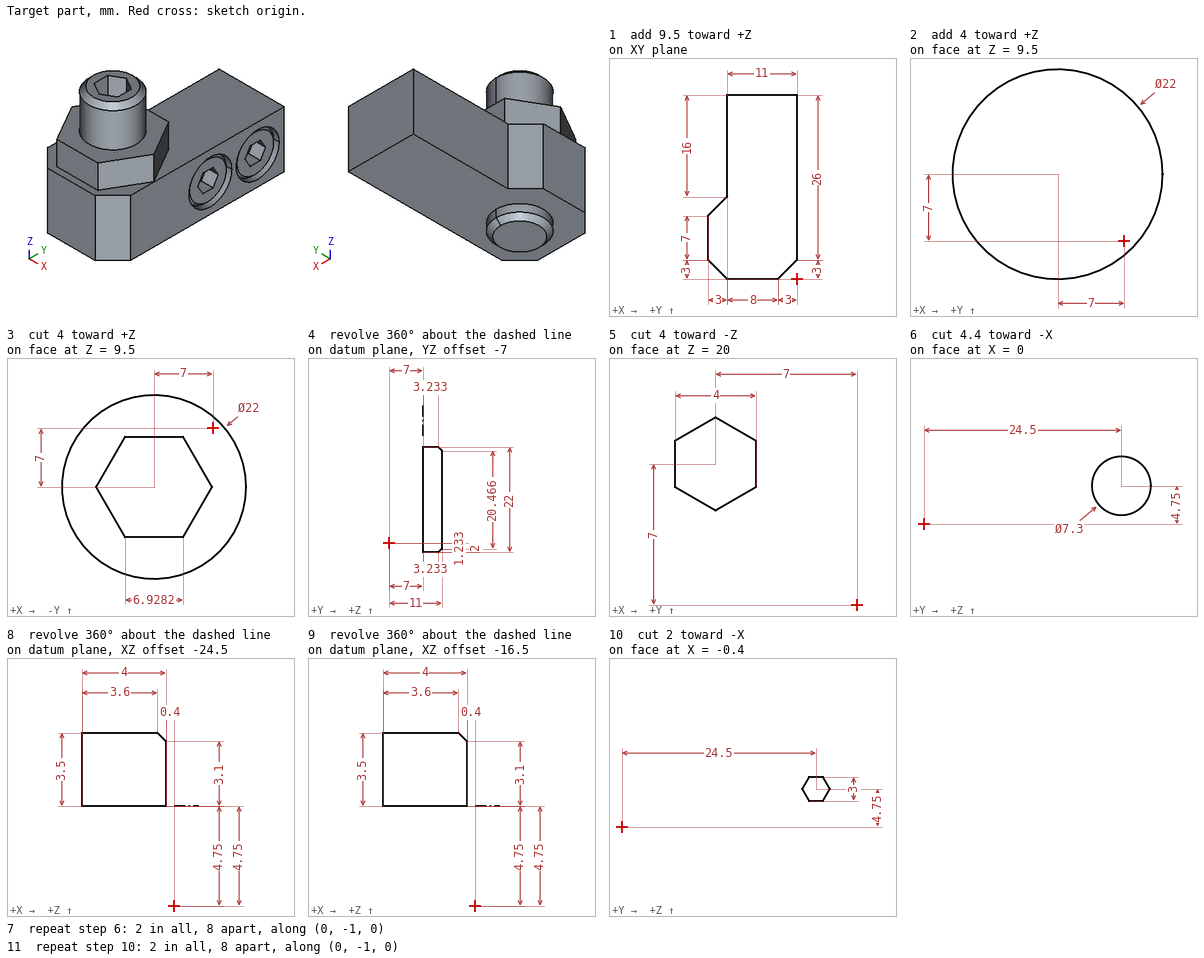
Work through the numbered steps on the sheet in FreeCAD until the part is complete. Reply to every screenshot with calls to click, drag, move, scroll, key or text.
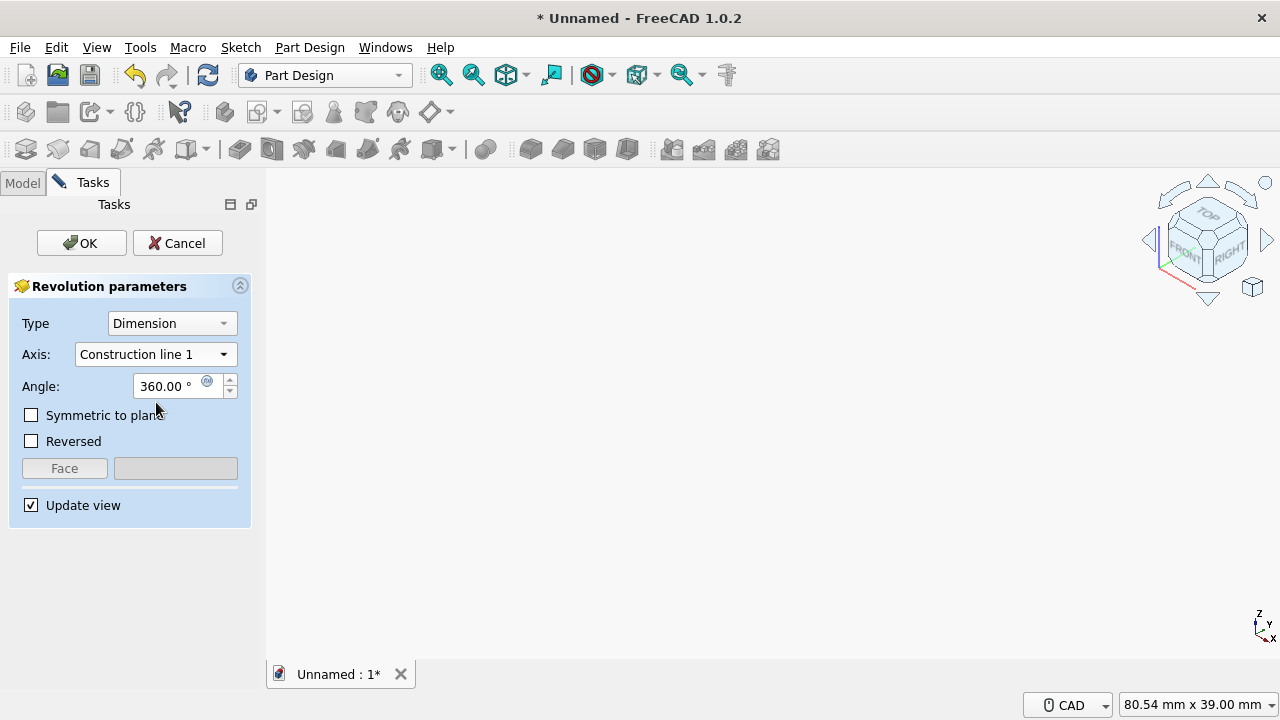
click(82, 243)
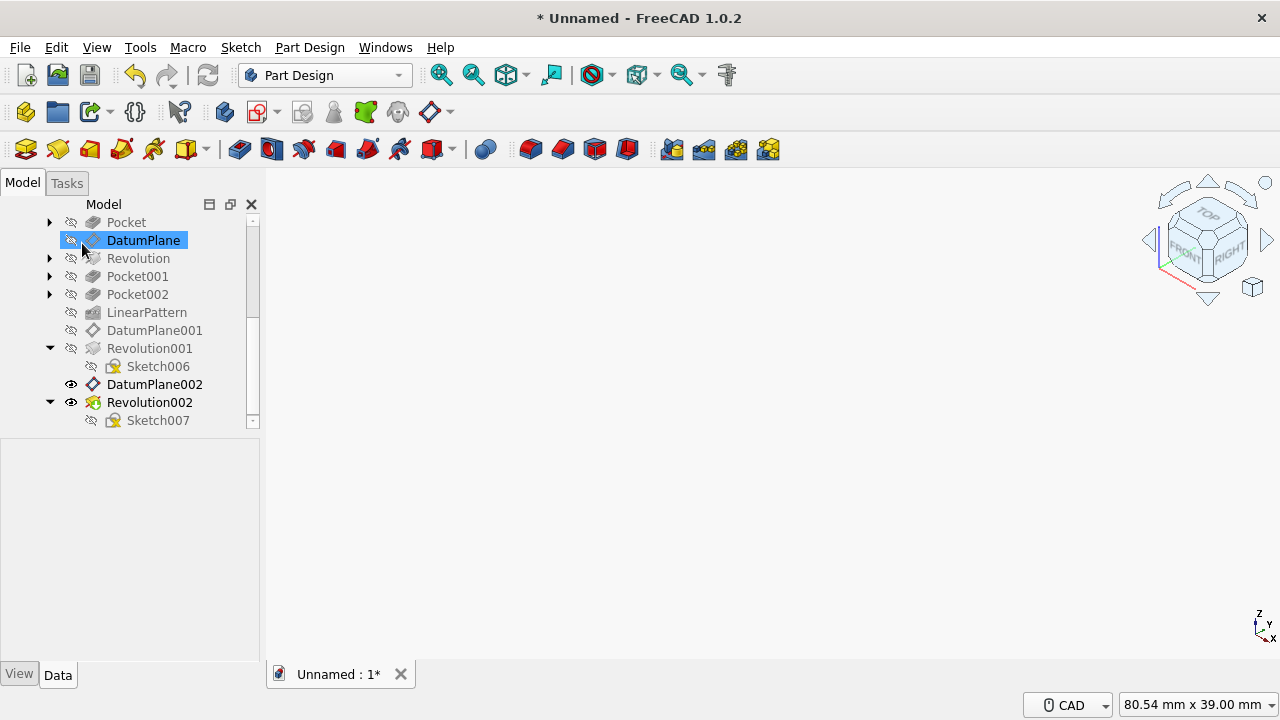
click(116, 384)
key(space)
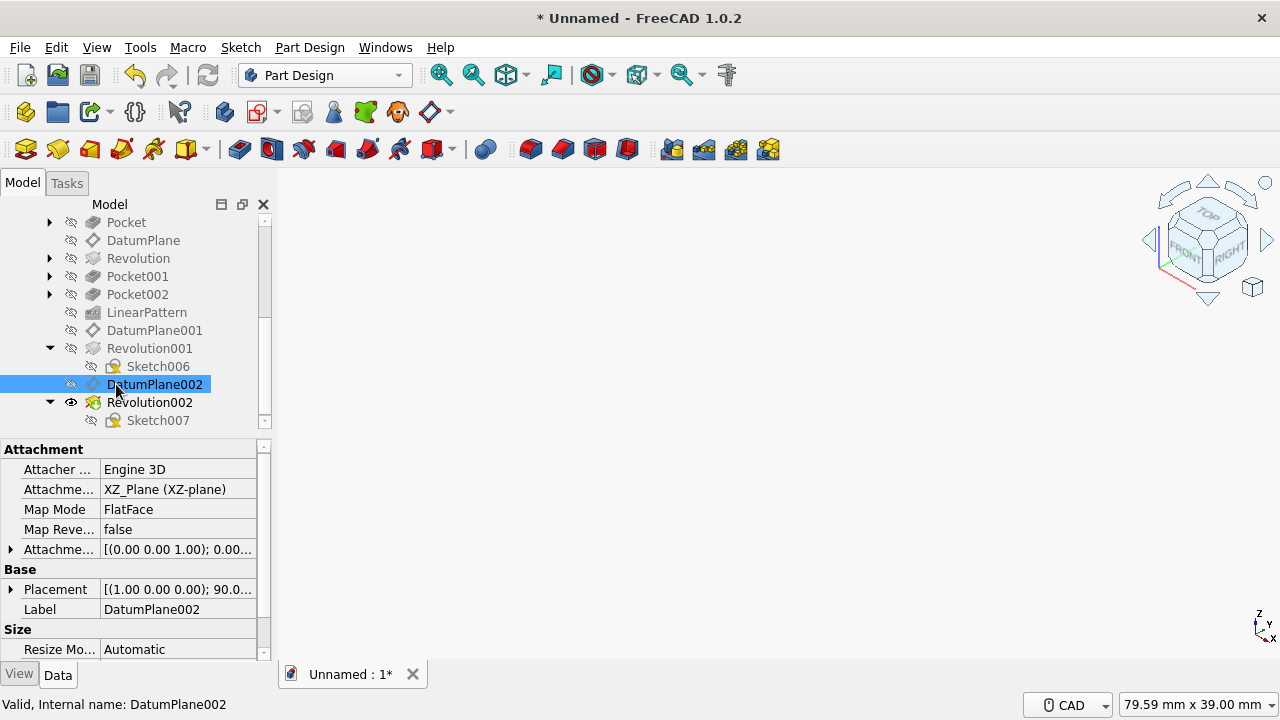
key(v)
key(f)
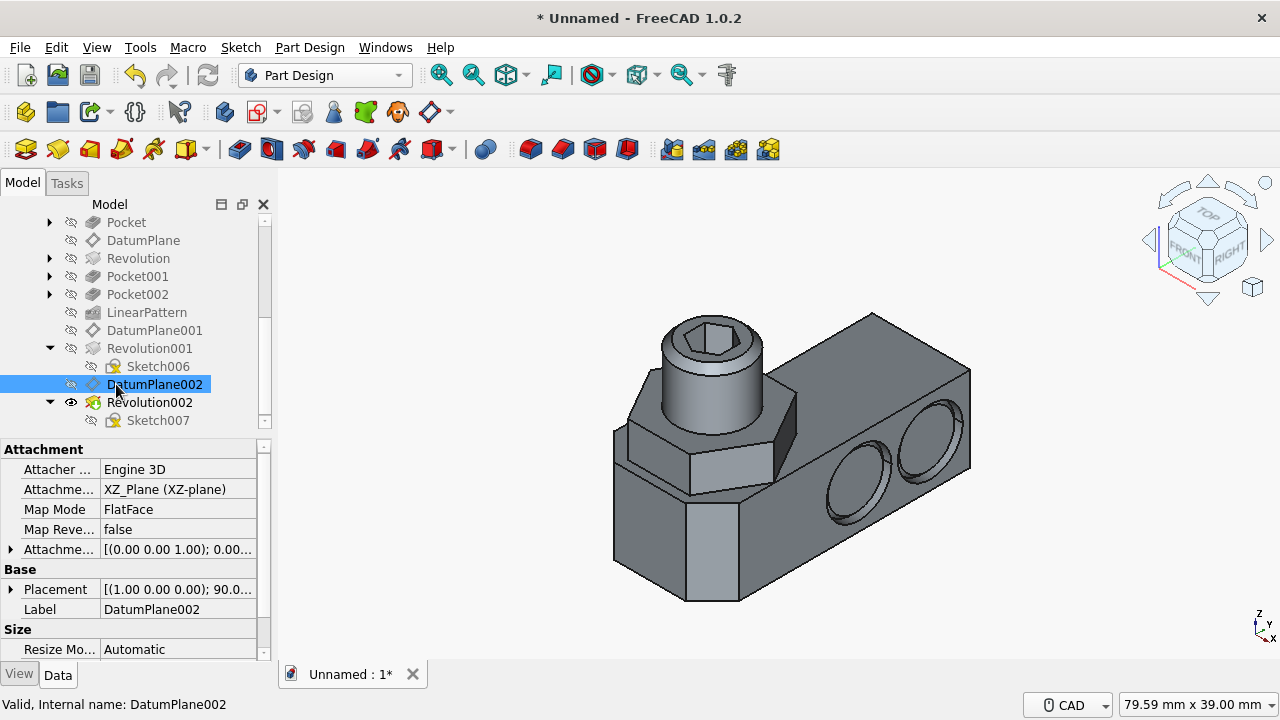
click(856, 480)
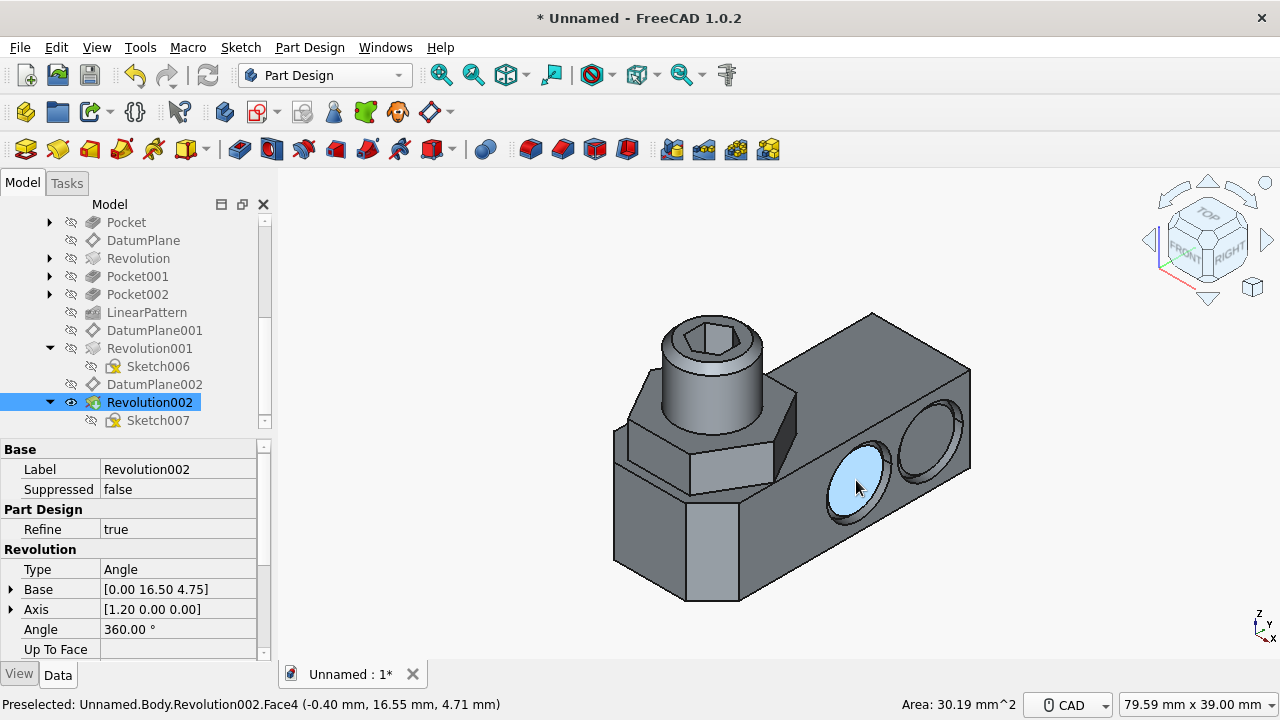
click(258, 112)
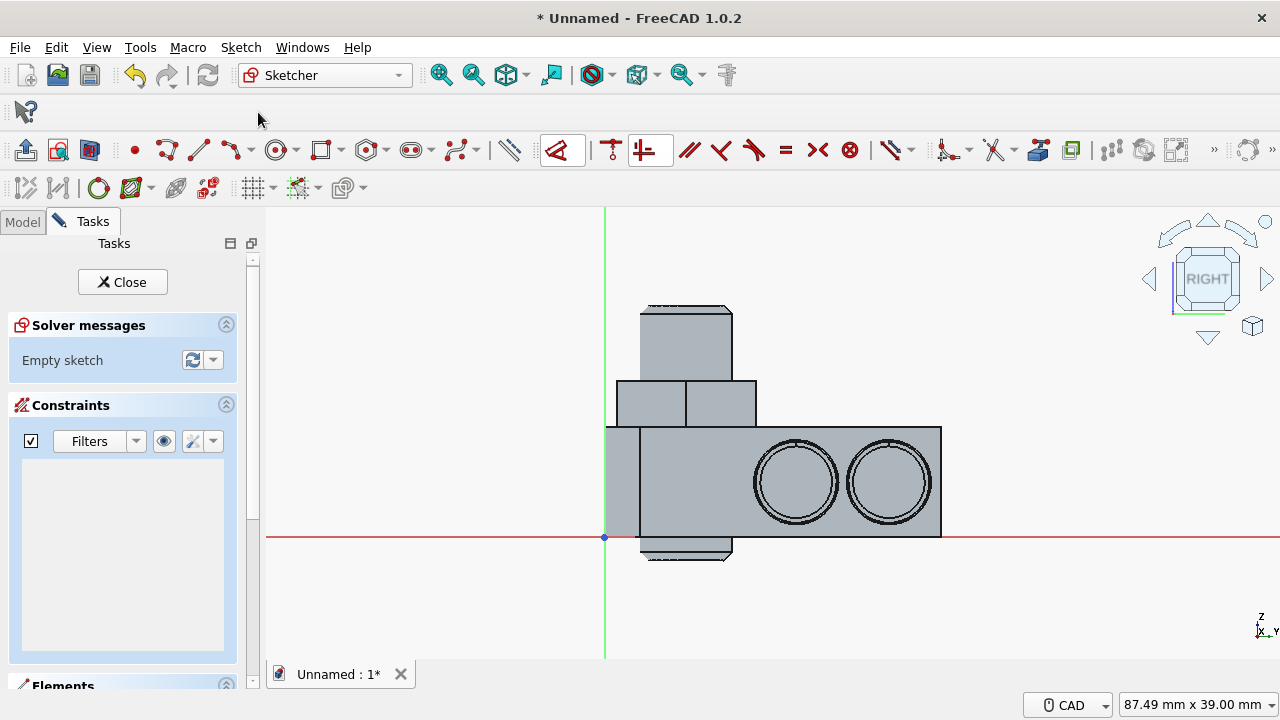
key(q)
key(s)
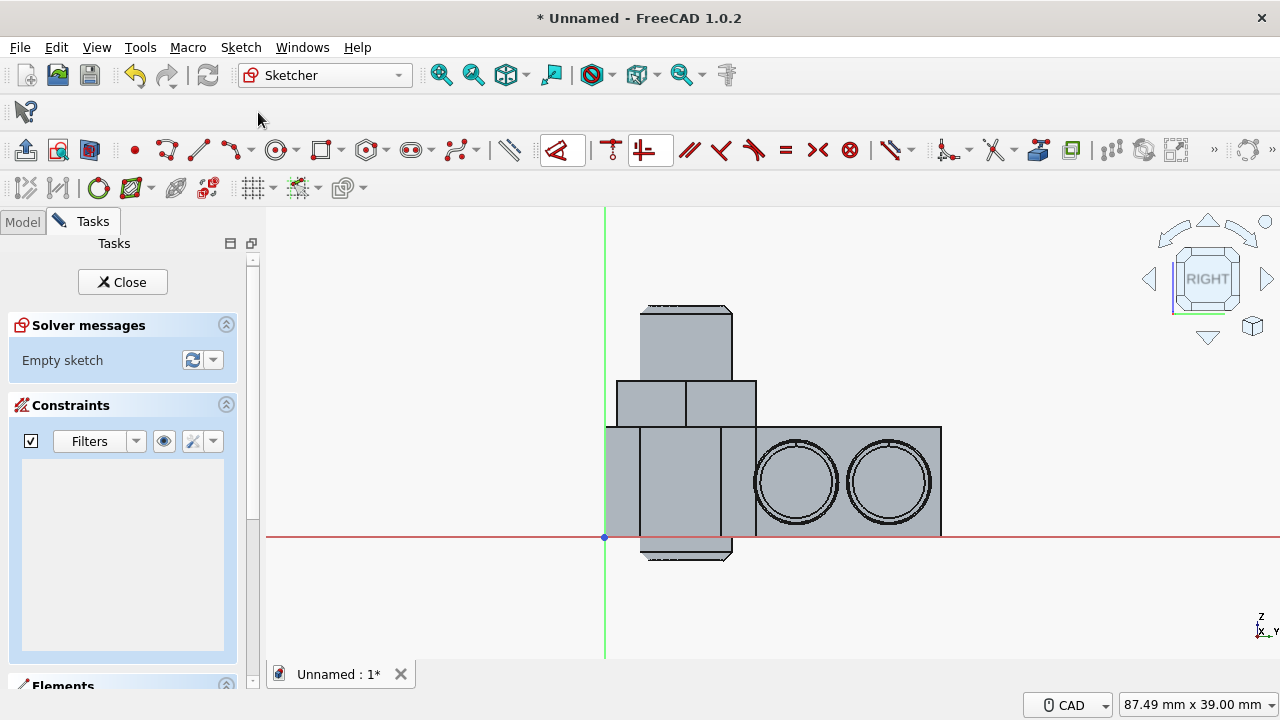
scroll(918, 490, up, 10)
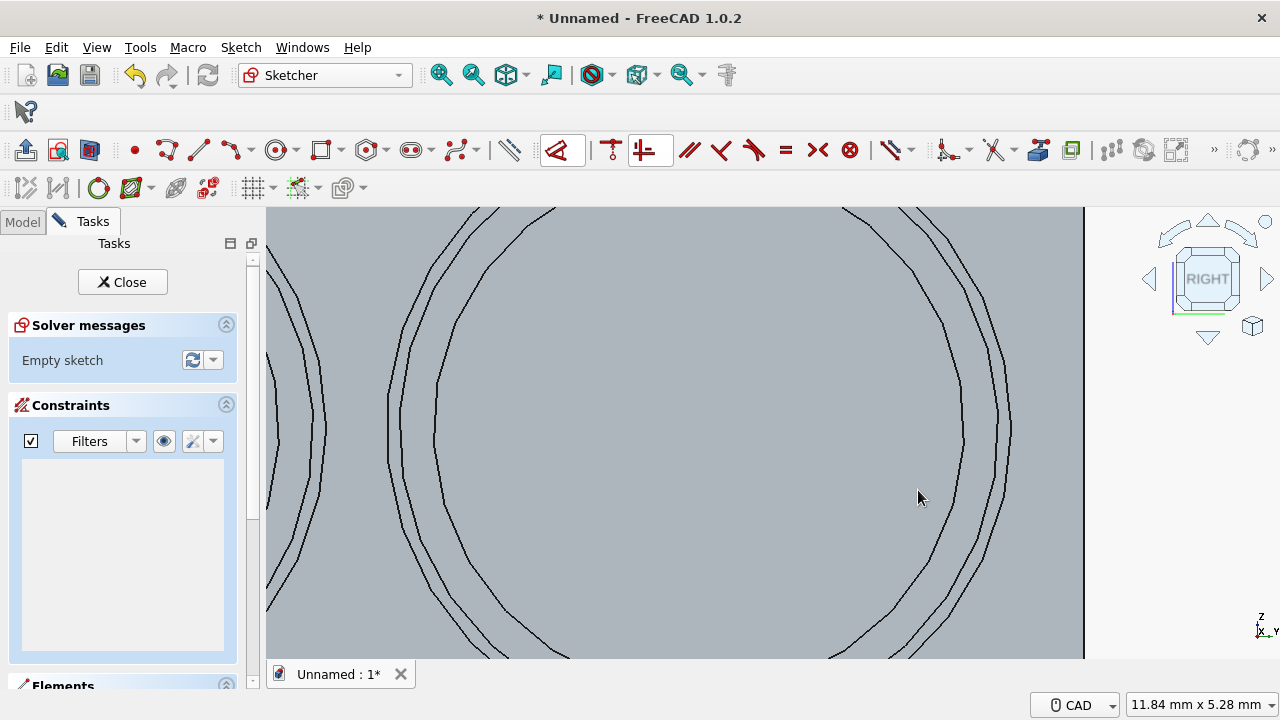
click(366, 150)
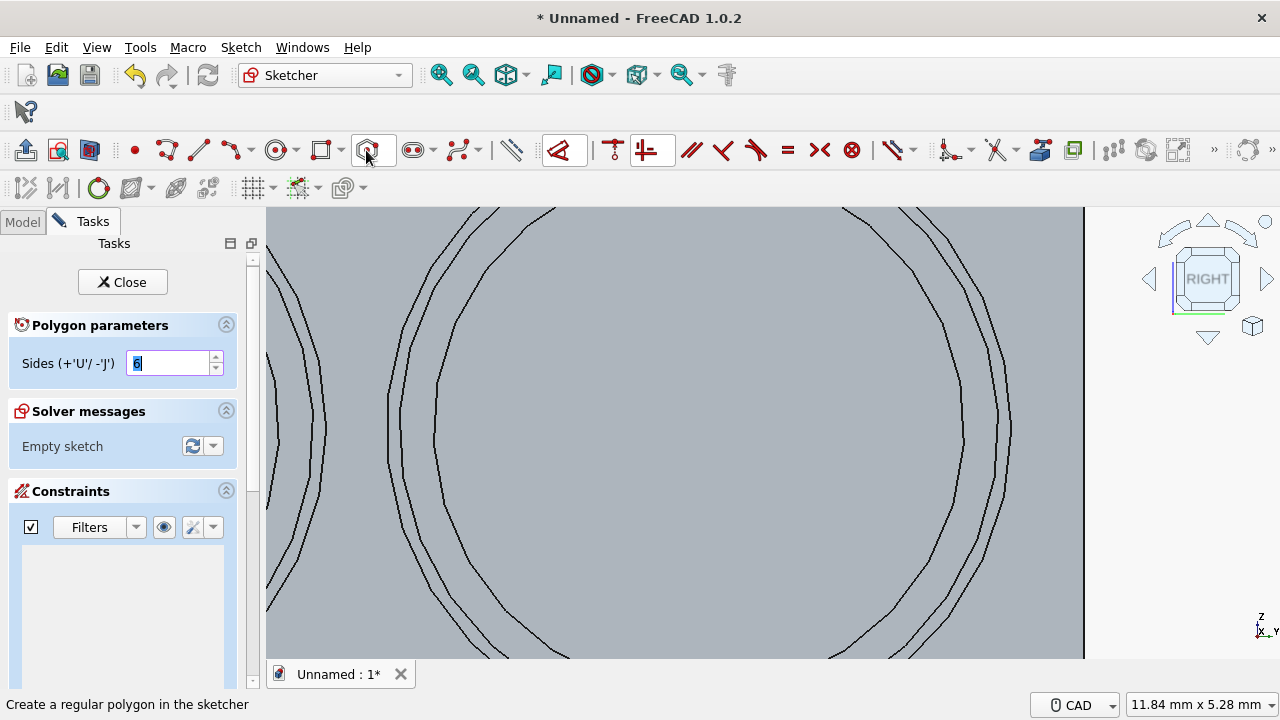
click(699, 429)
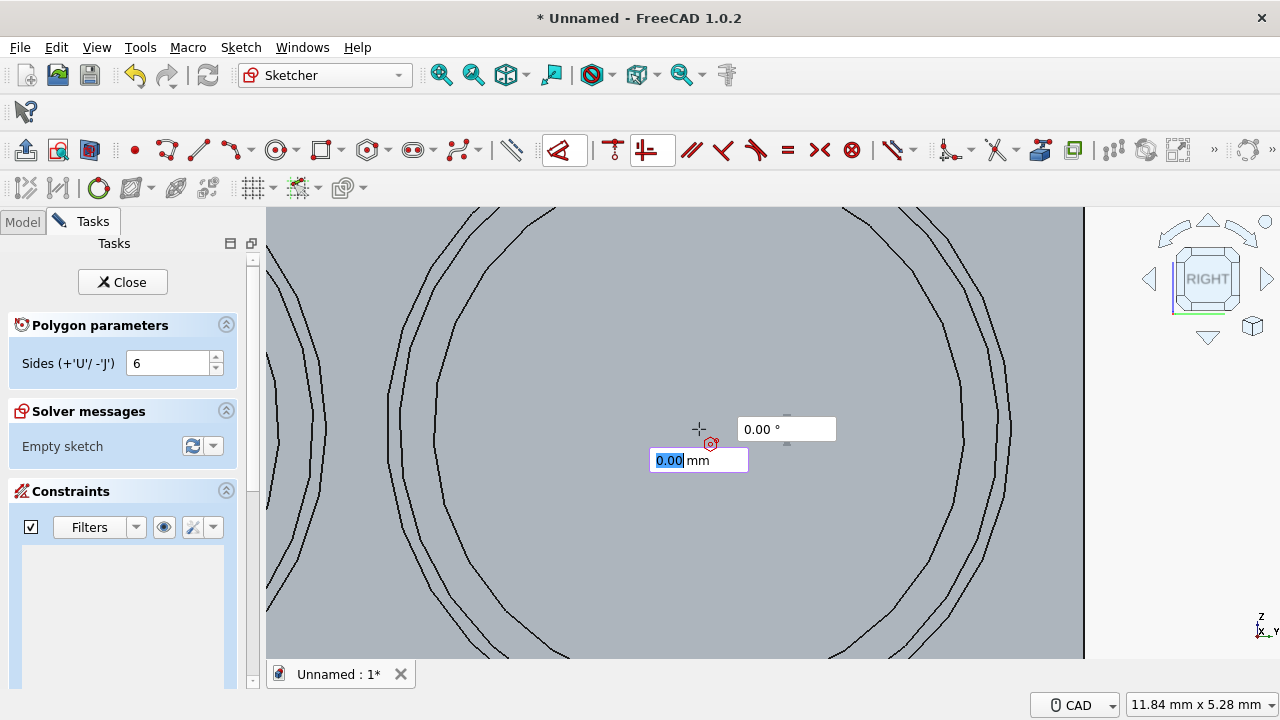
click(551, 429)
right_click(551, 429)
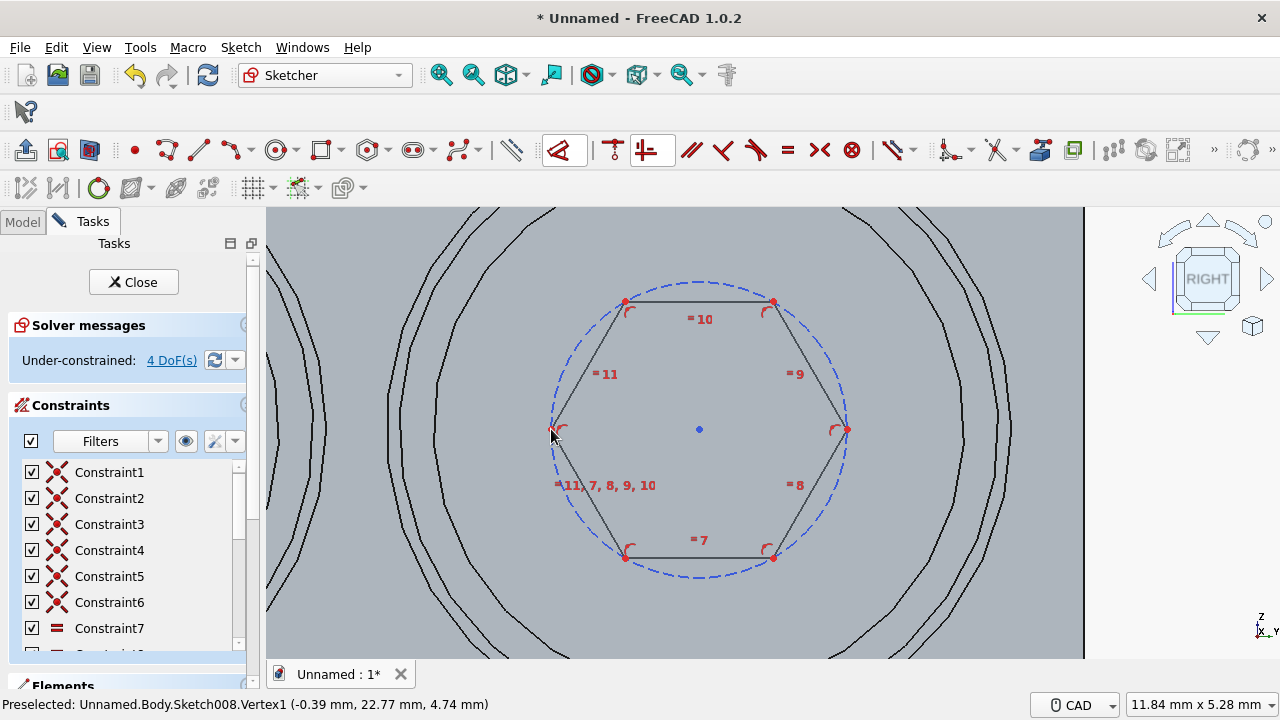
click(669, 558)